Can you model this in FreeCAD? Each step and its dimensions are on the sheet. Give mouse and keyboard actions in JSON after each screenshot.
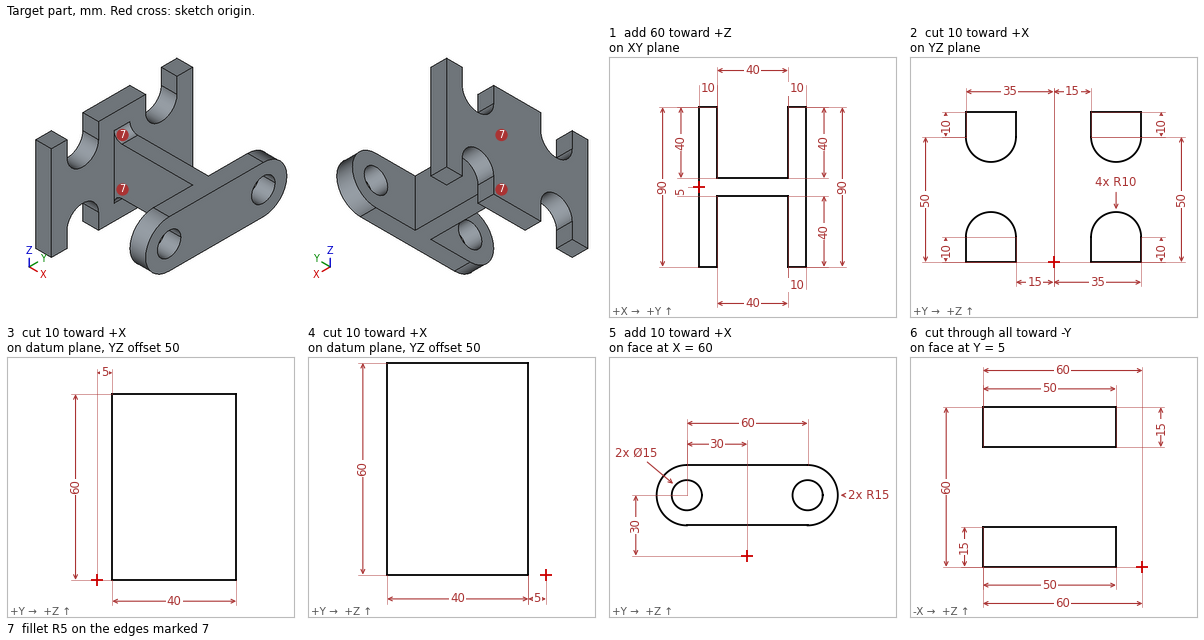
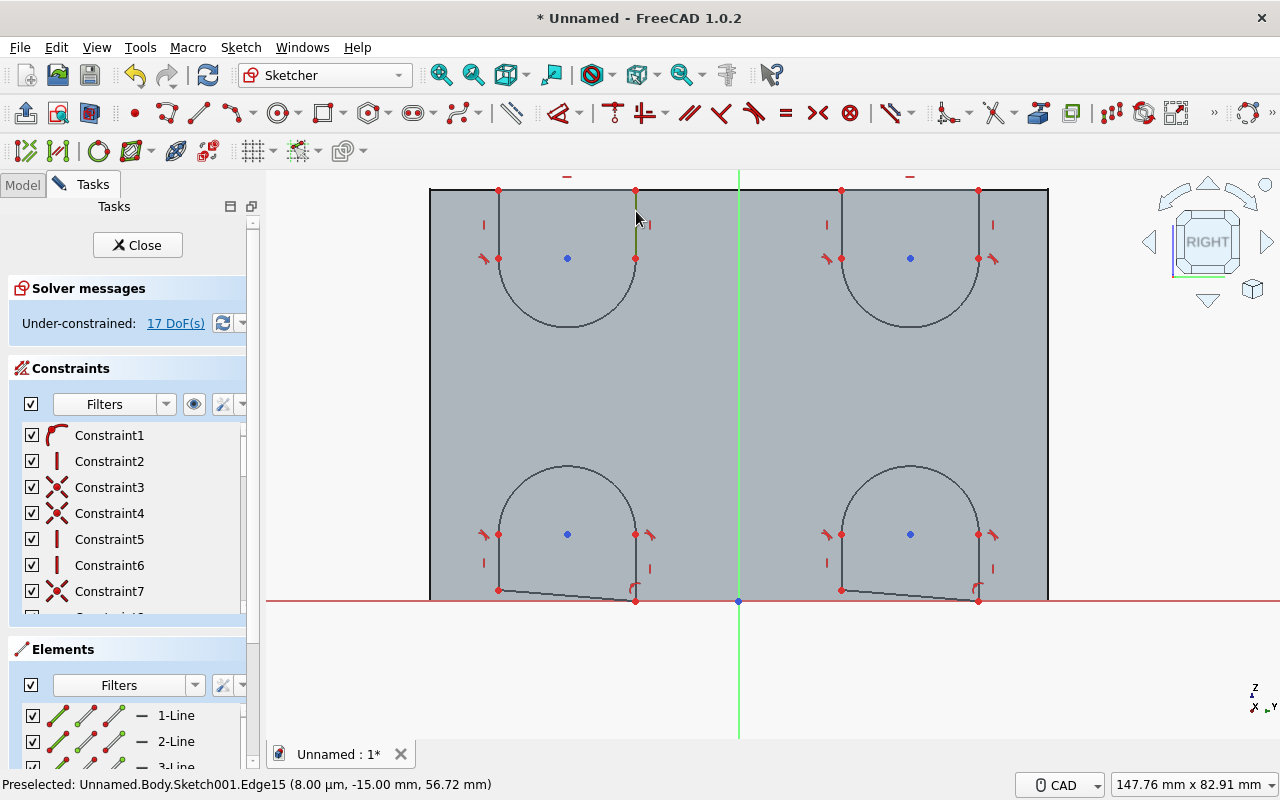
{"action": "left_click", "coordinate": [527, 314]}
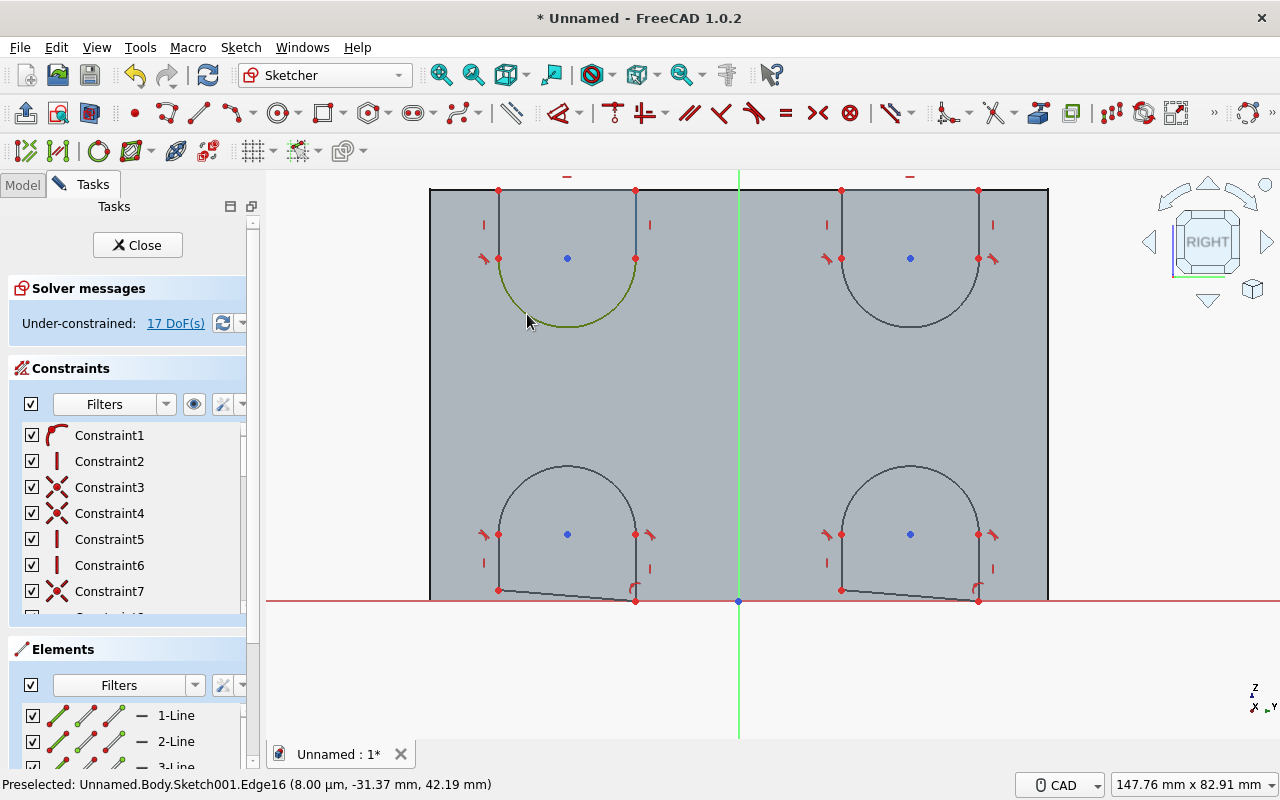
{"action": "left_click", "coordinate": [754, 114]}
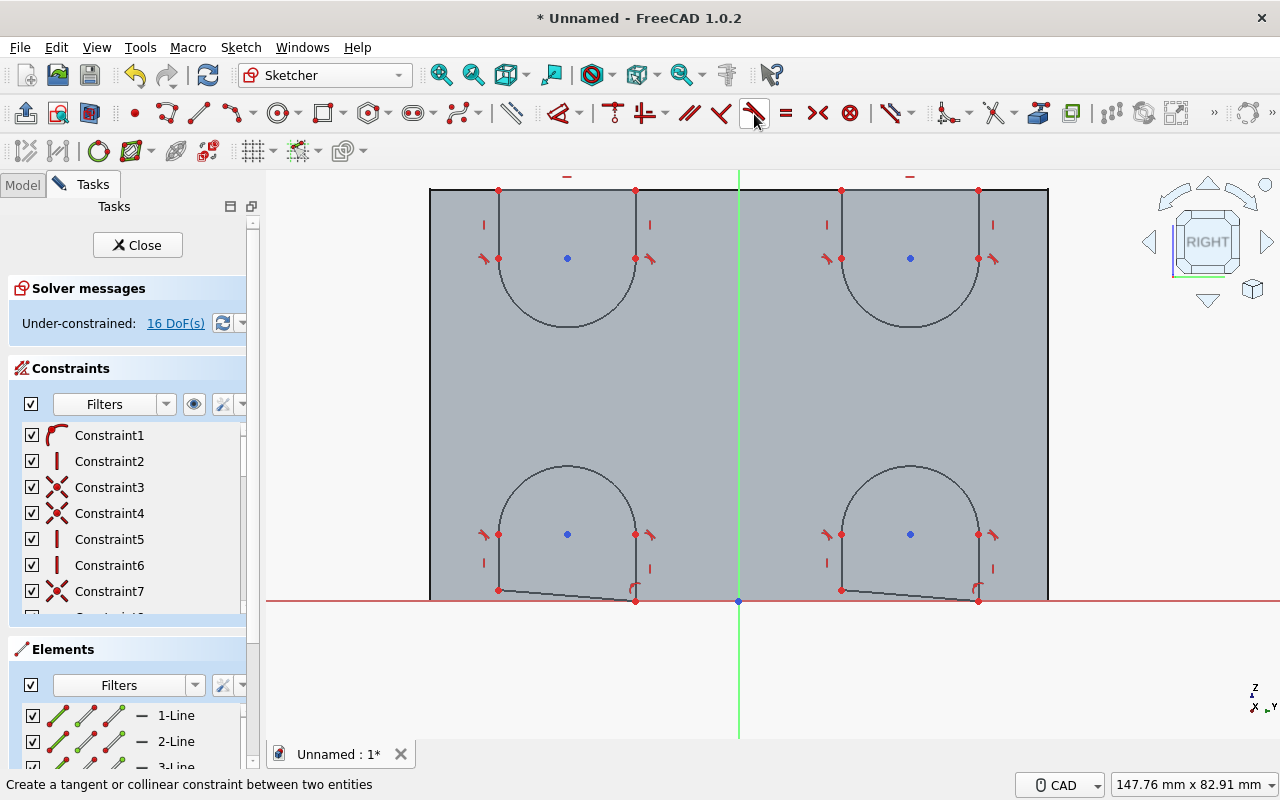
{"action": "left_click", "coordinate": [938, 598]}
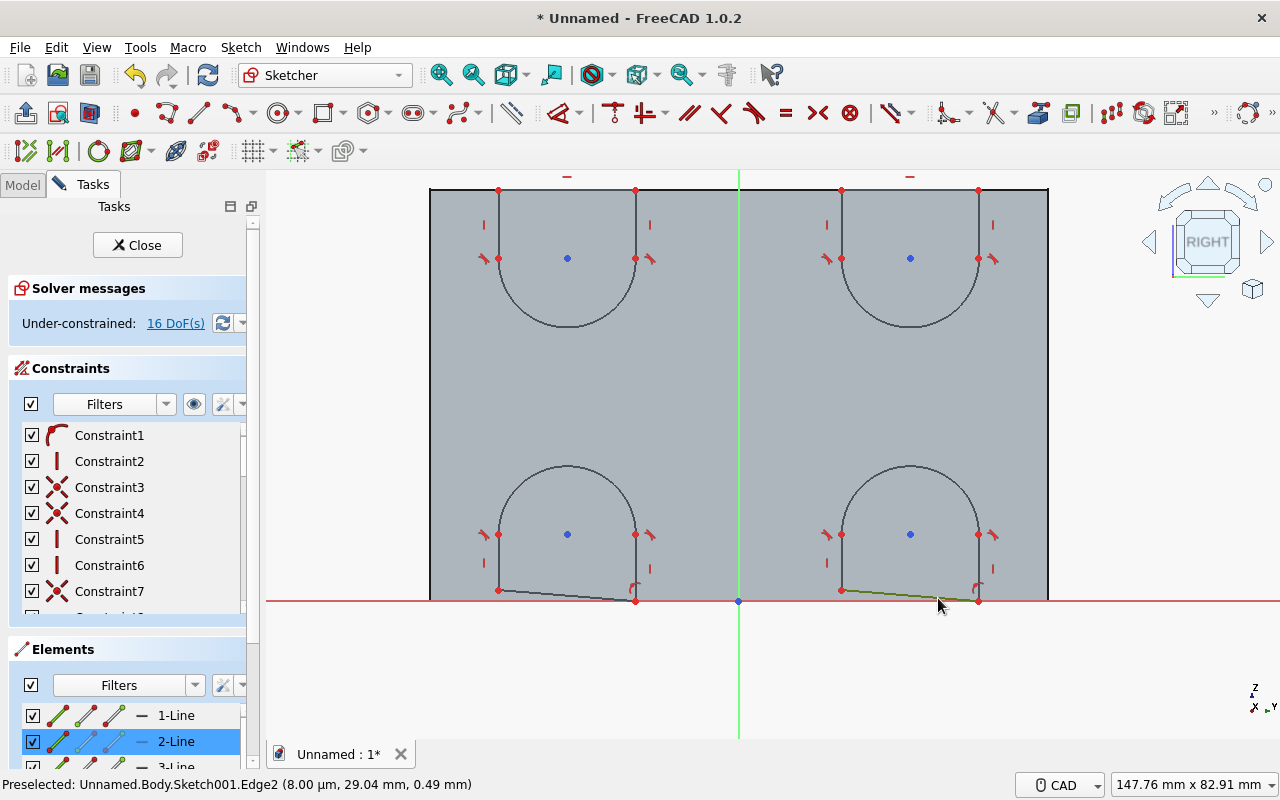
{"action": "left_click", "coordinate": [668, 114]}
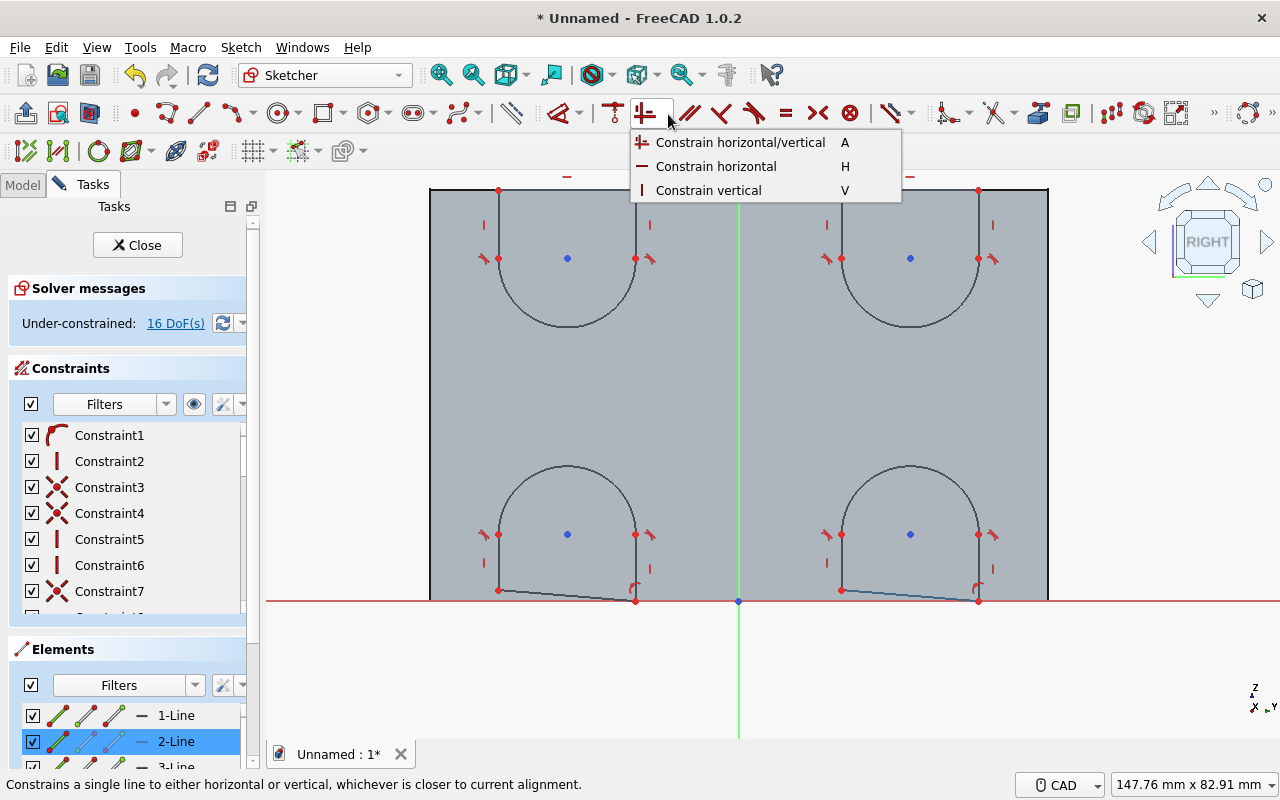
{"action": "left_click", "coordinate": [766, 166]}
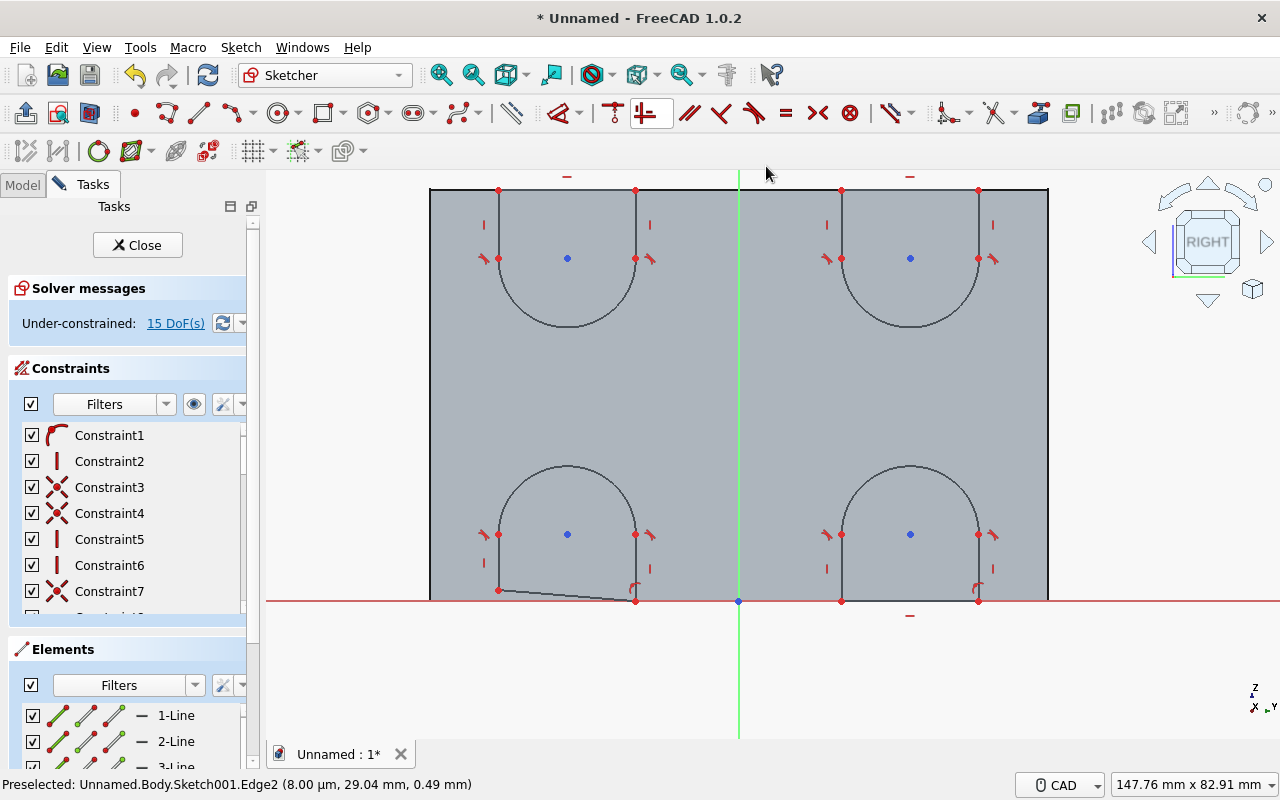
{"action": "left_click", "coordinate": [595, 598]}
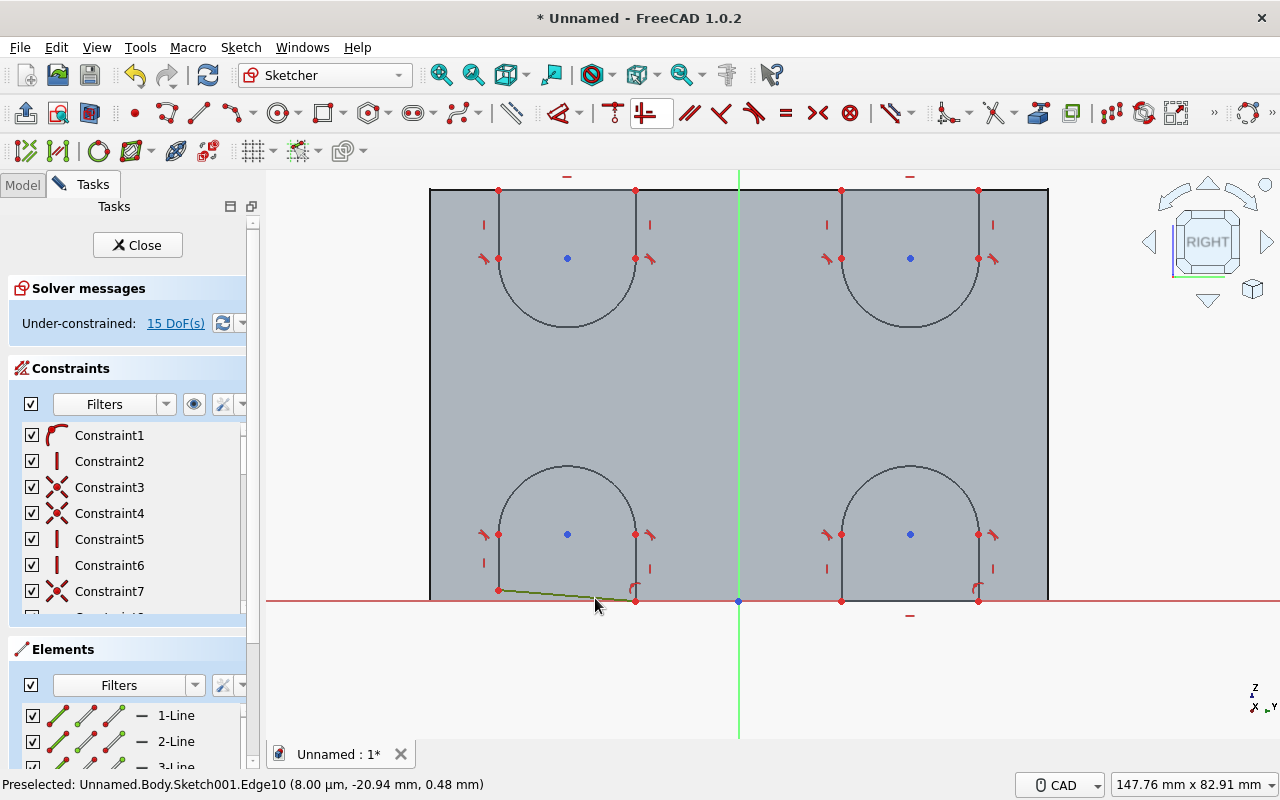
{"action": "left_click", "coordinate": [668, 114]}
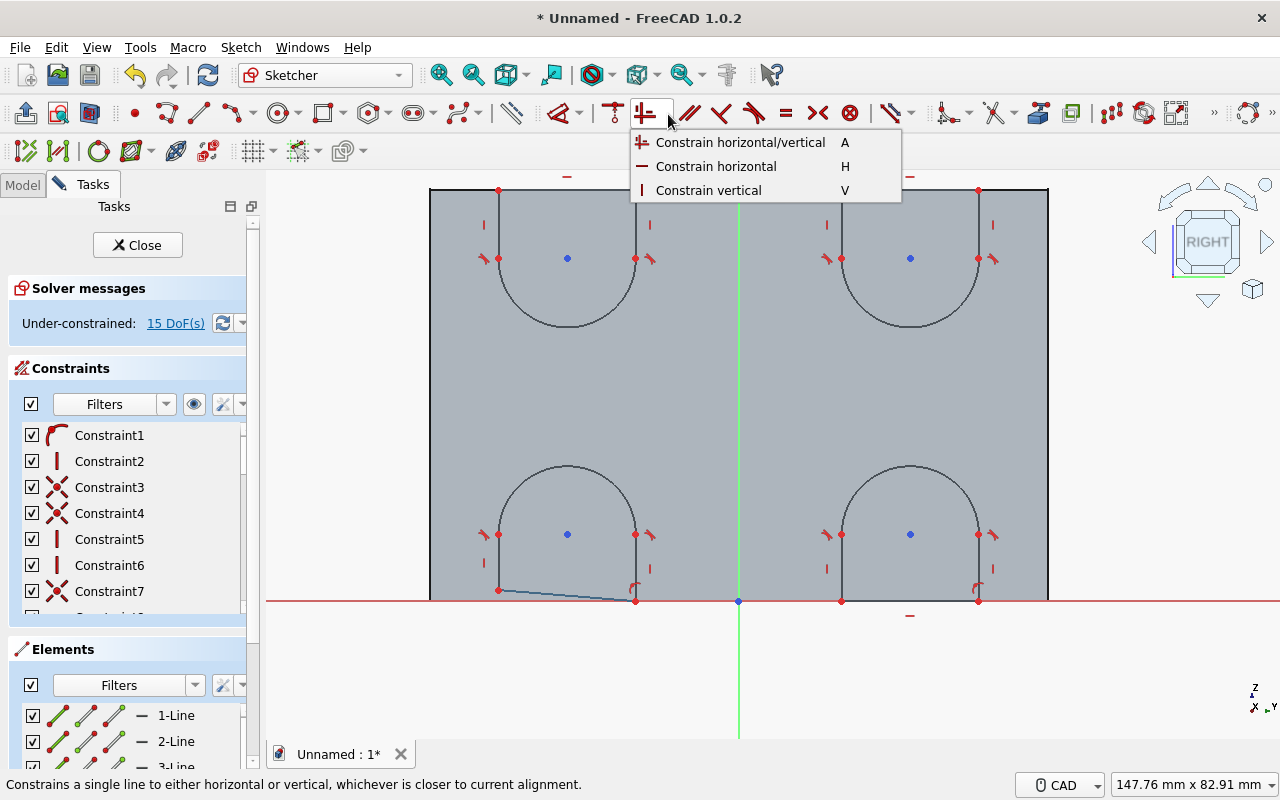
{"action": "left_click", "coordinate": [766, 166]}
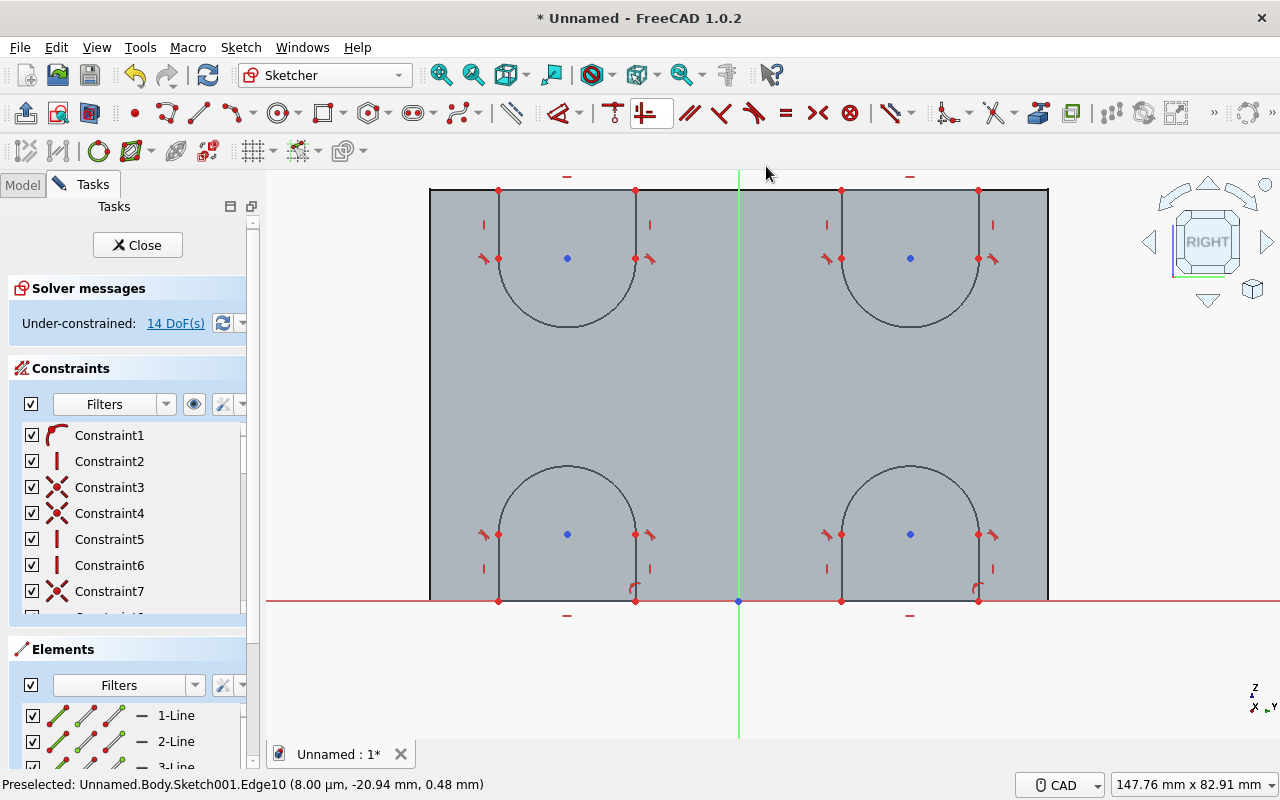
{"action": "left_click", "coordinate": [951, 479]}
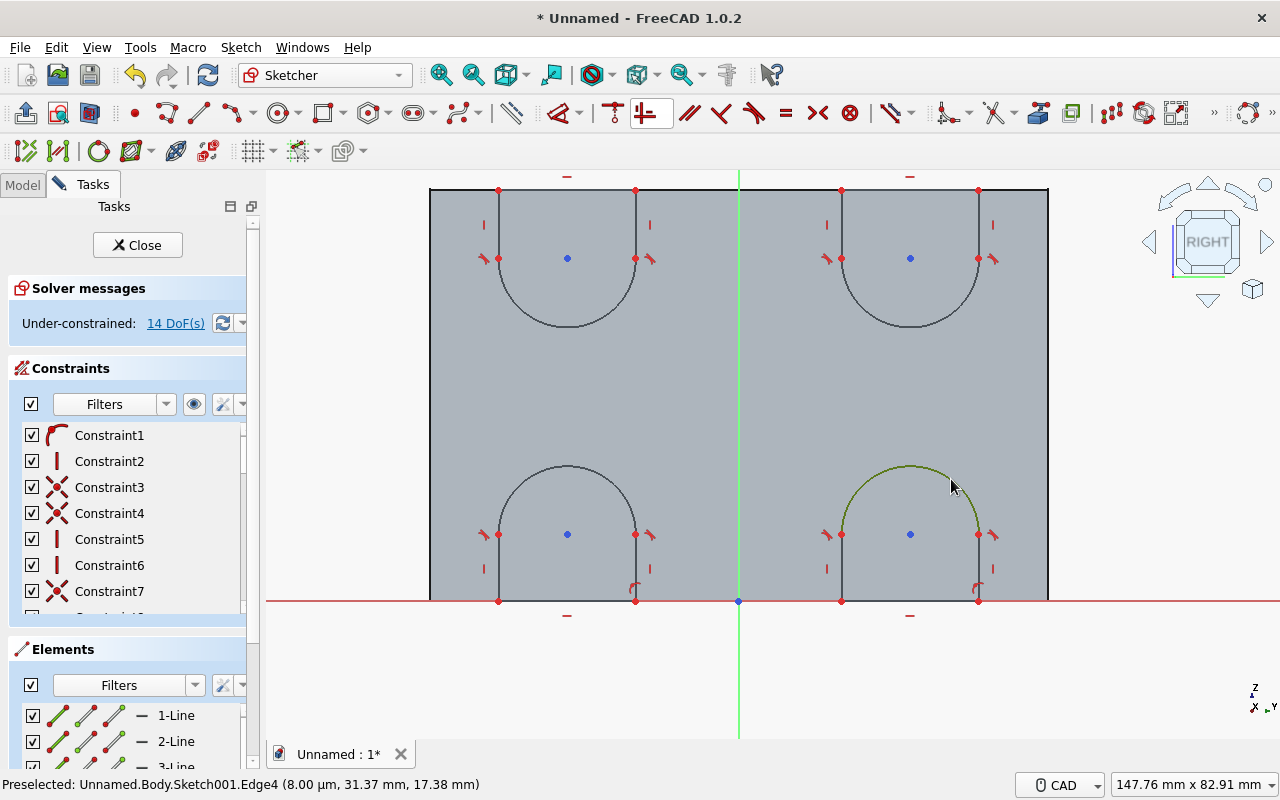
{"action": "left_click", "coordinate": [870, 314]}